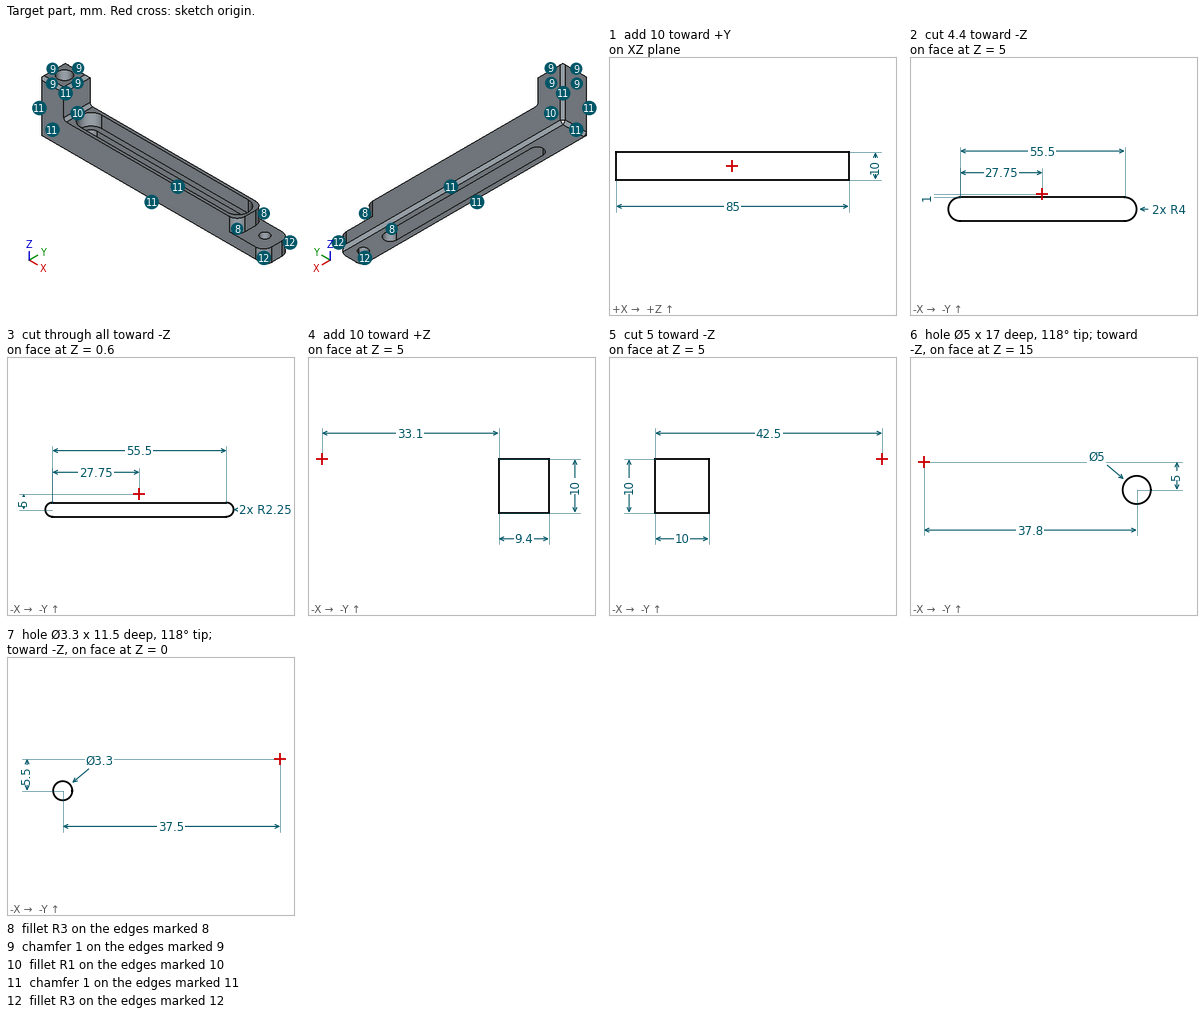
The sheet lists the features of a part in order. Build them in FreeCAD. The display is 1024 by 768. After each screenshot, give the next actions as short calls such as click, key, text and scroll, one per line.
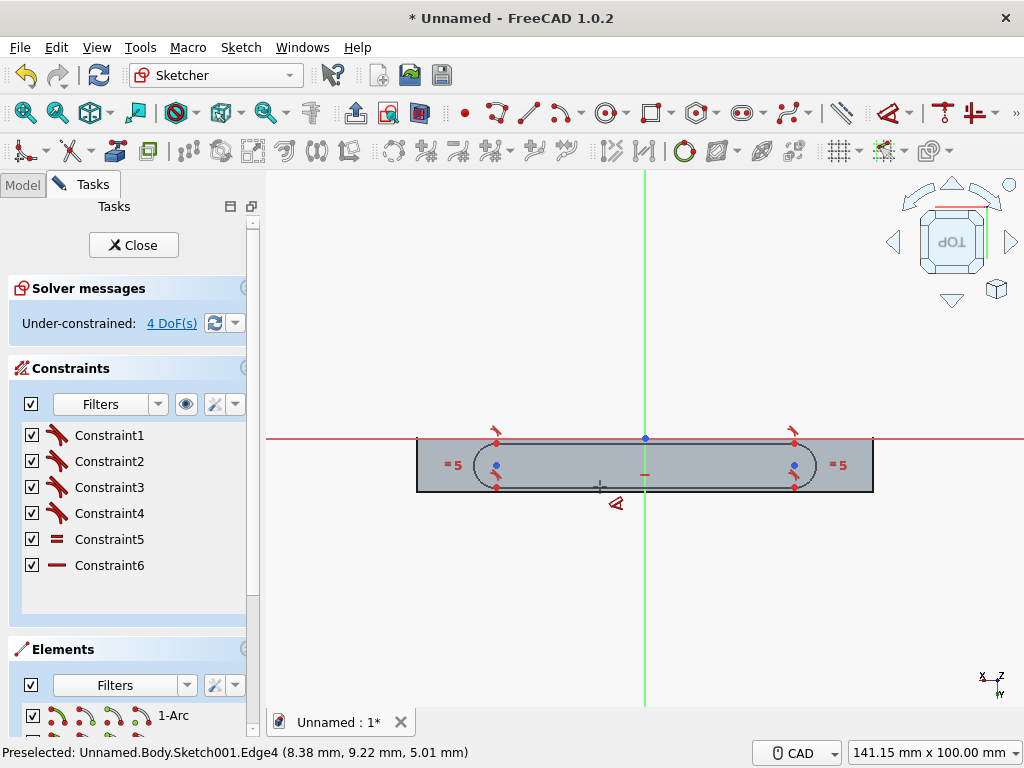
scroll(478, 453, up, 4)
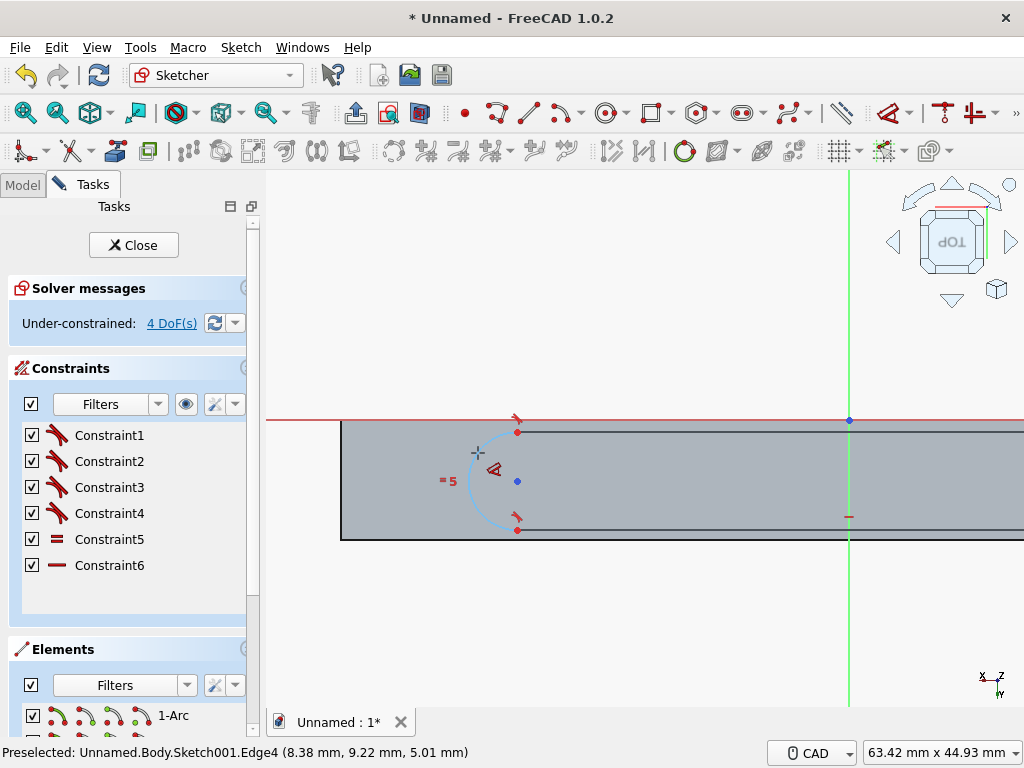
click(478, 453)
click(452, 434)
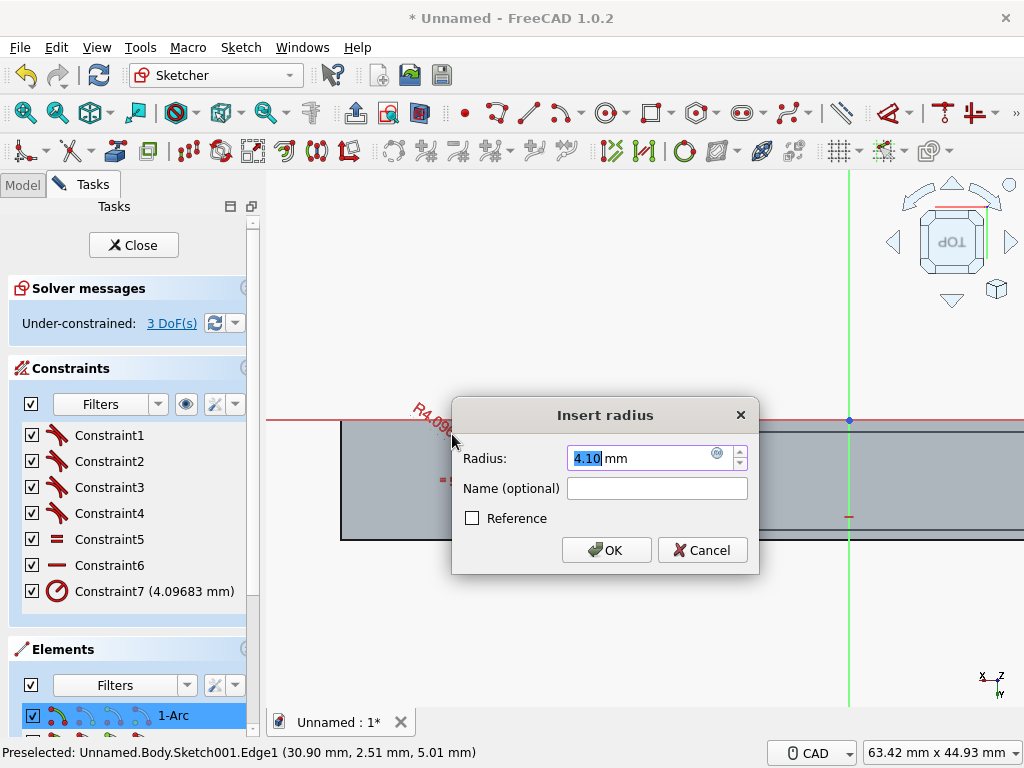
text(4)
key(Return)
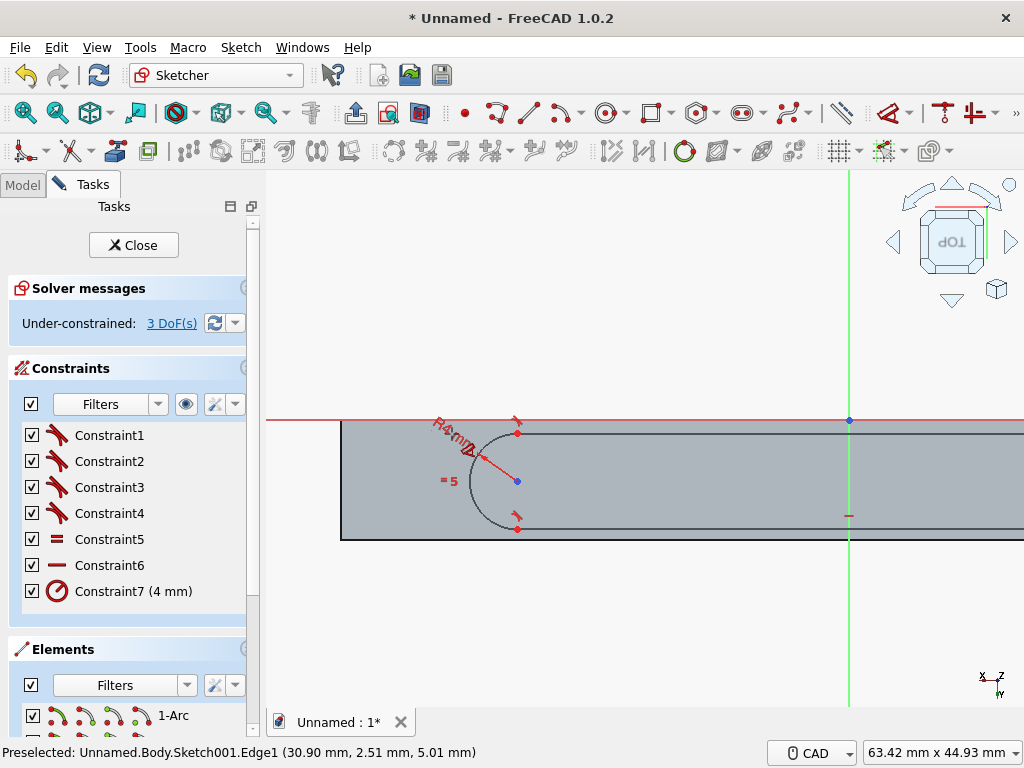
scroll(518, 434, up, 7)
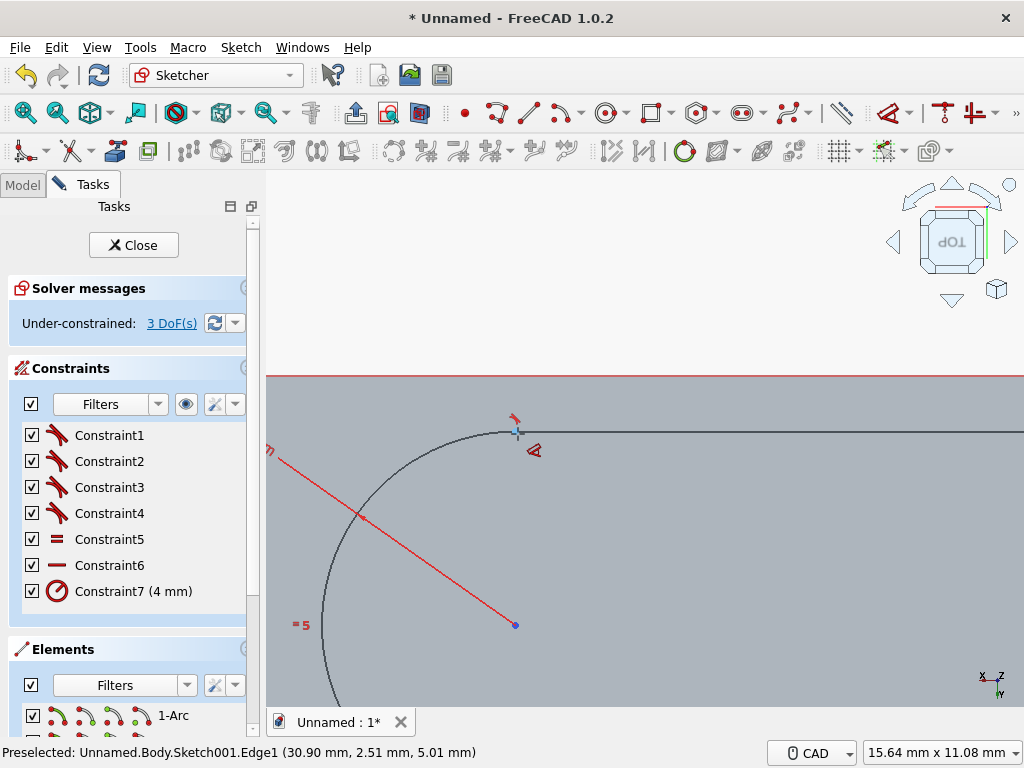
click(516, 432)
click(482, 404)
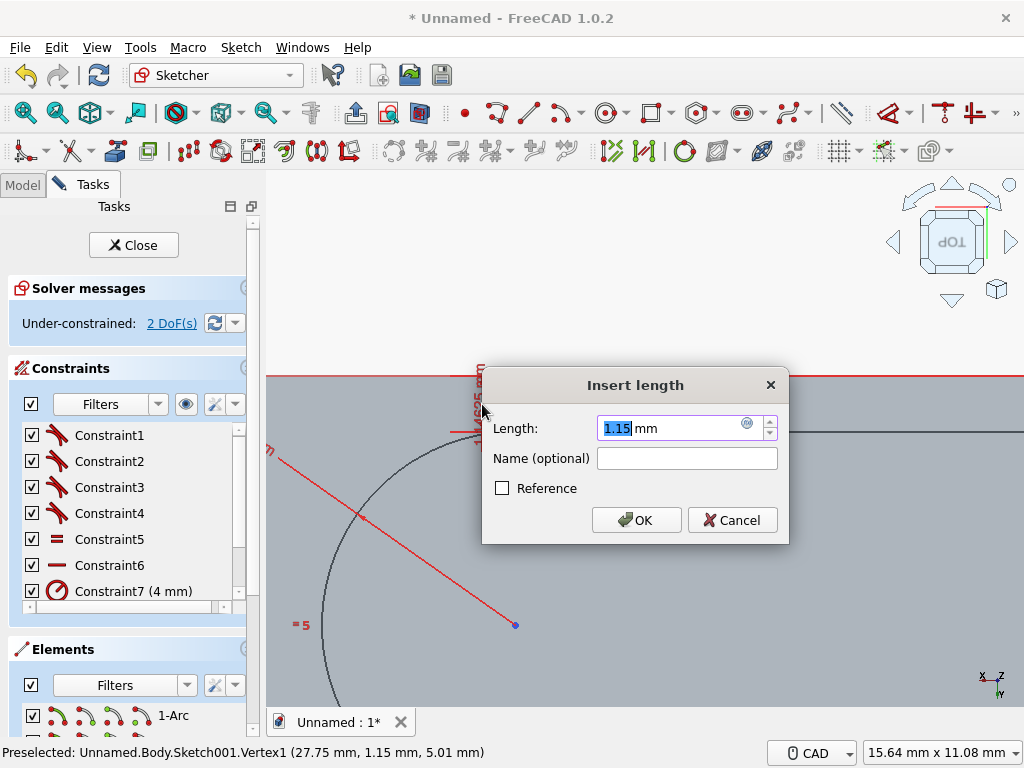
text(1)
key(Return)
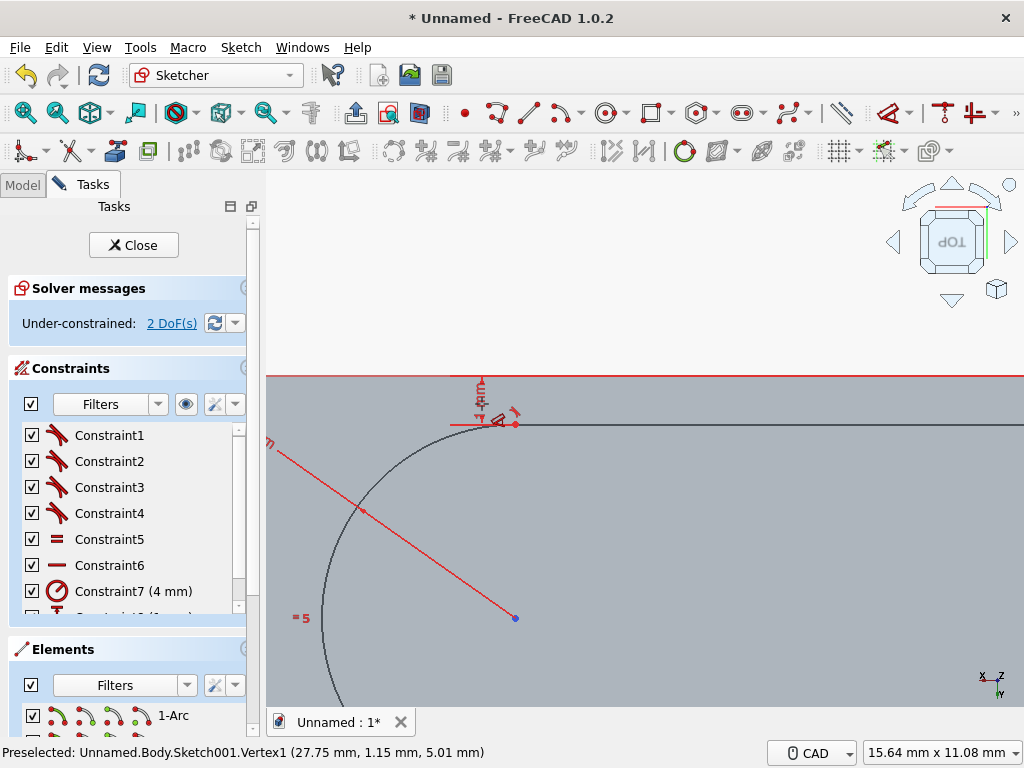
scroll(376, 414, down, 10)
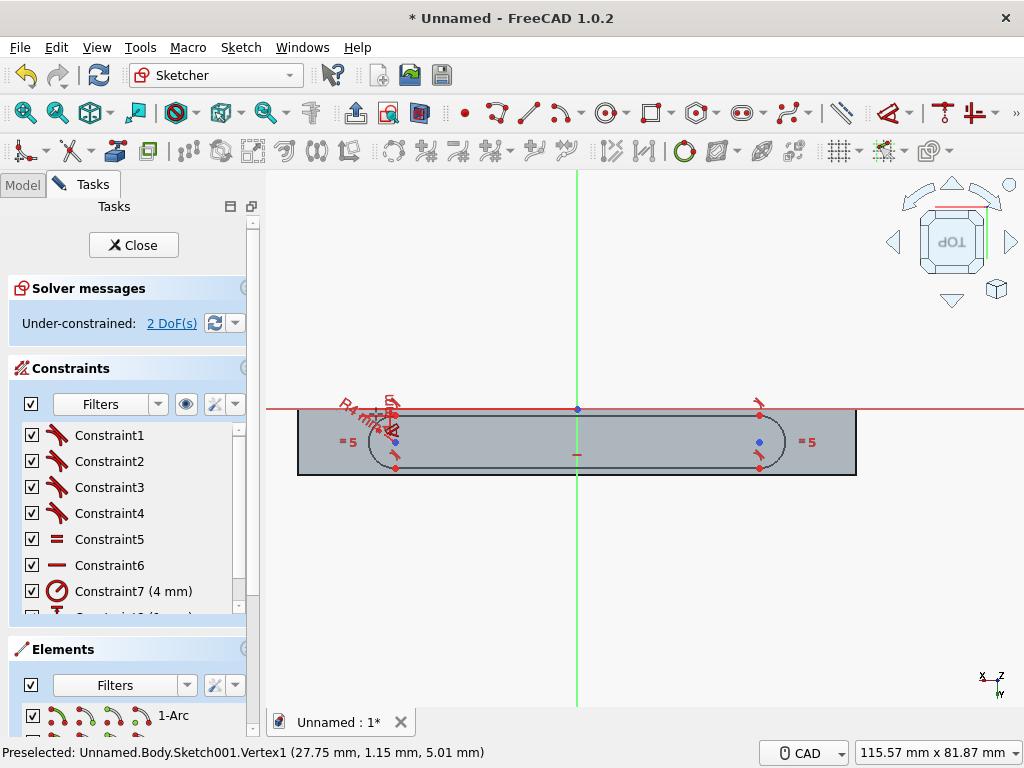
scroll(504, 416, up, 4)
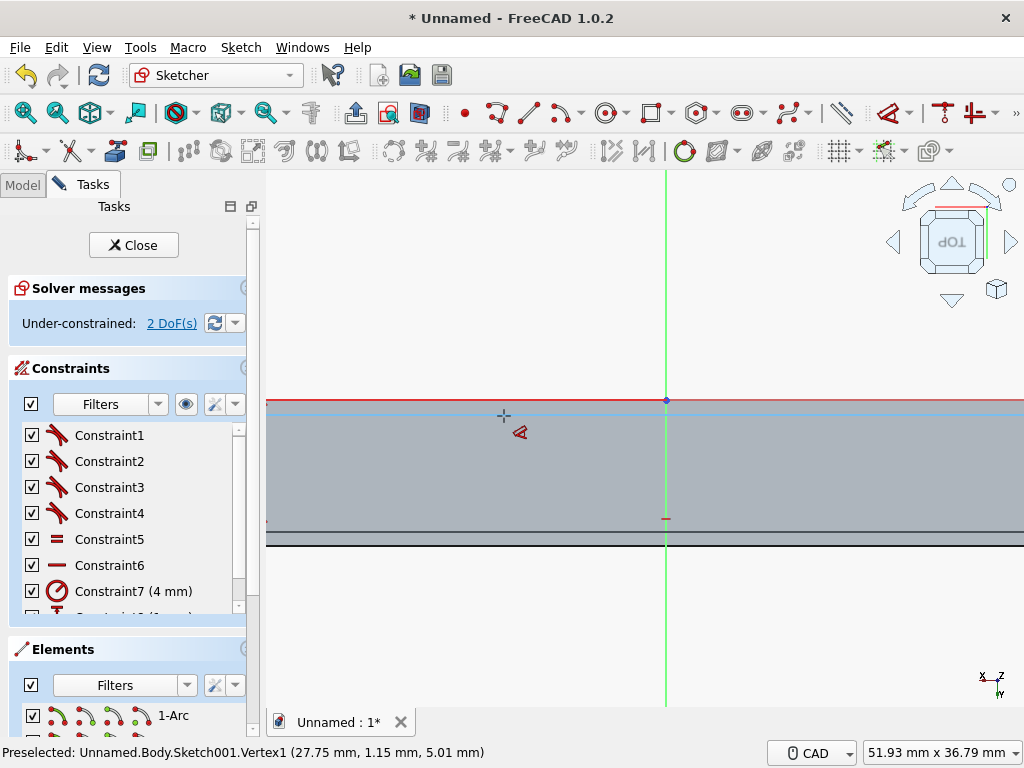
click(504, 415)
click(576, 381)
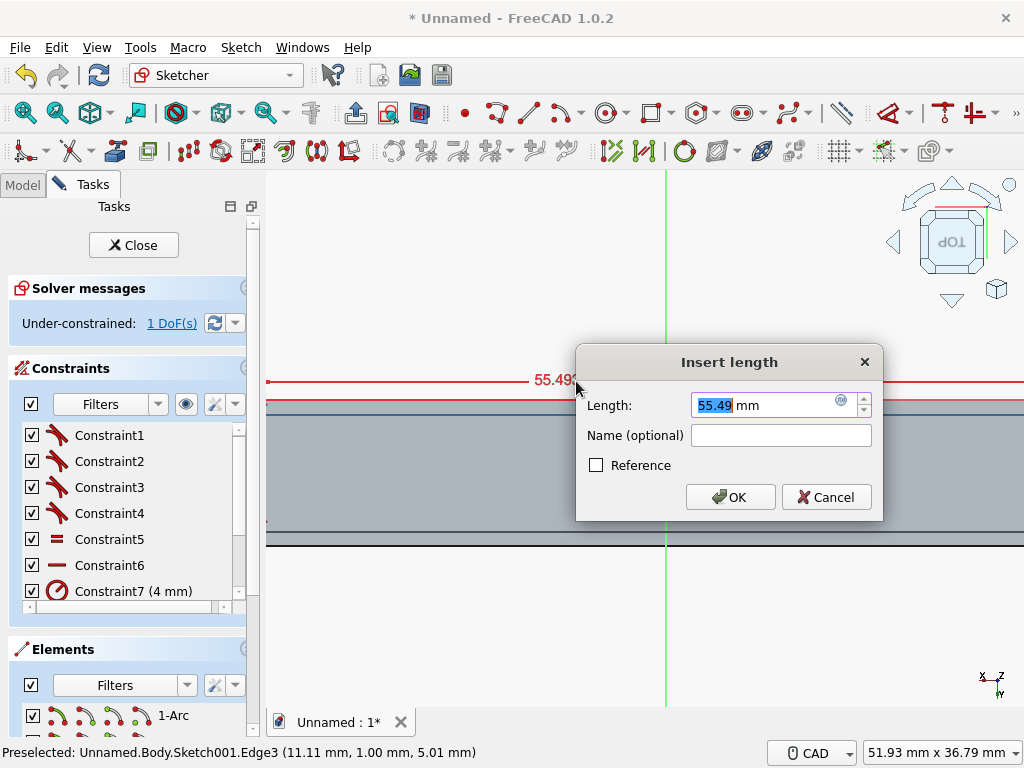
text(55.5)
key(Return)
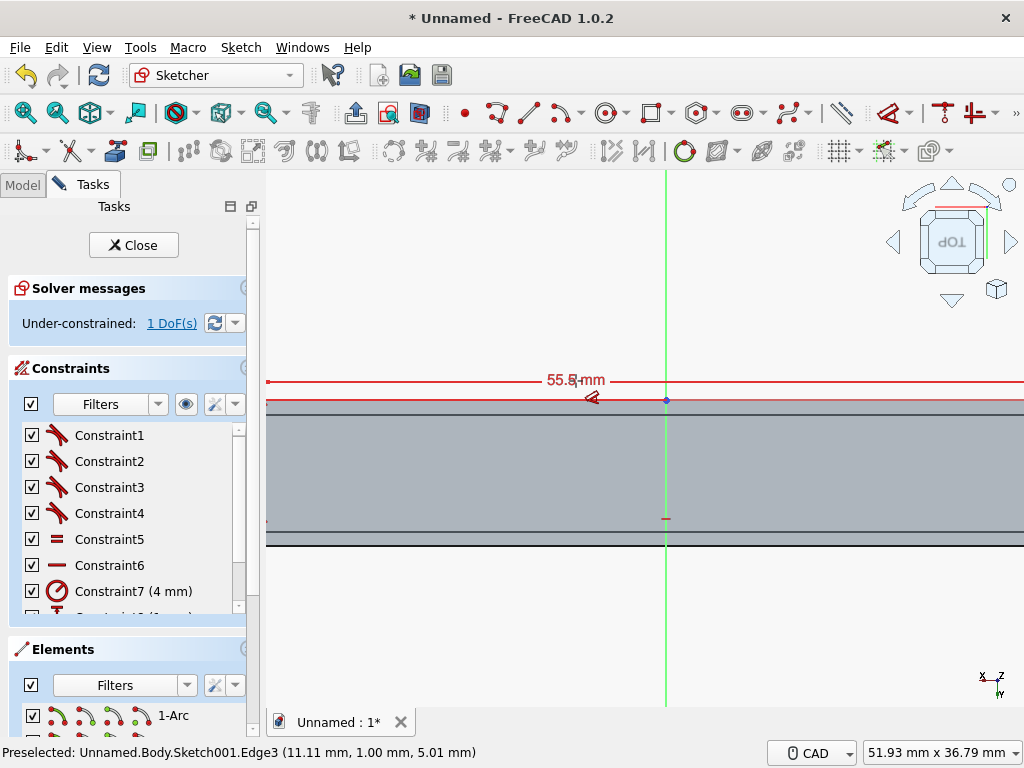
scroll(503, 416, down, 4)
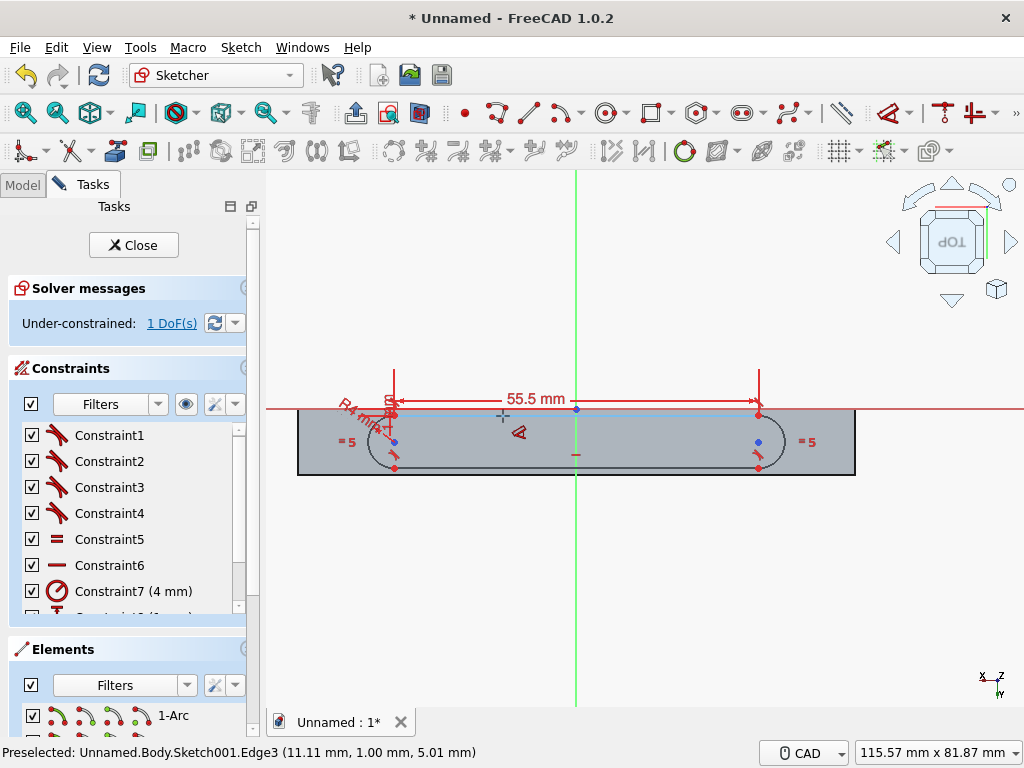
click(394, 416)
click(485, 375)